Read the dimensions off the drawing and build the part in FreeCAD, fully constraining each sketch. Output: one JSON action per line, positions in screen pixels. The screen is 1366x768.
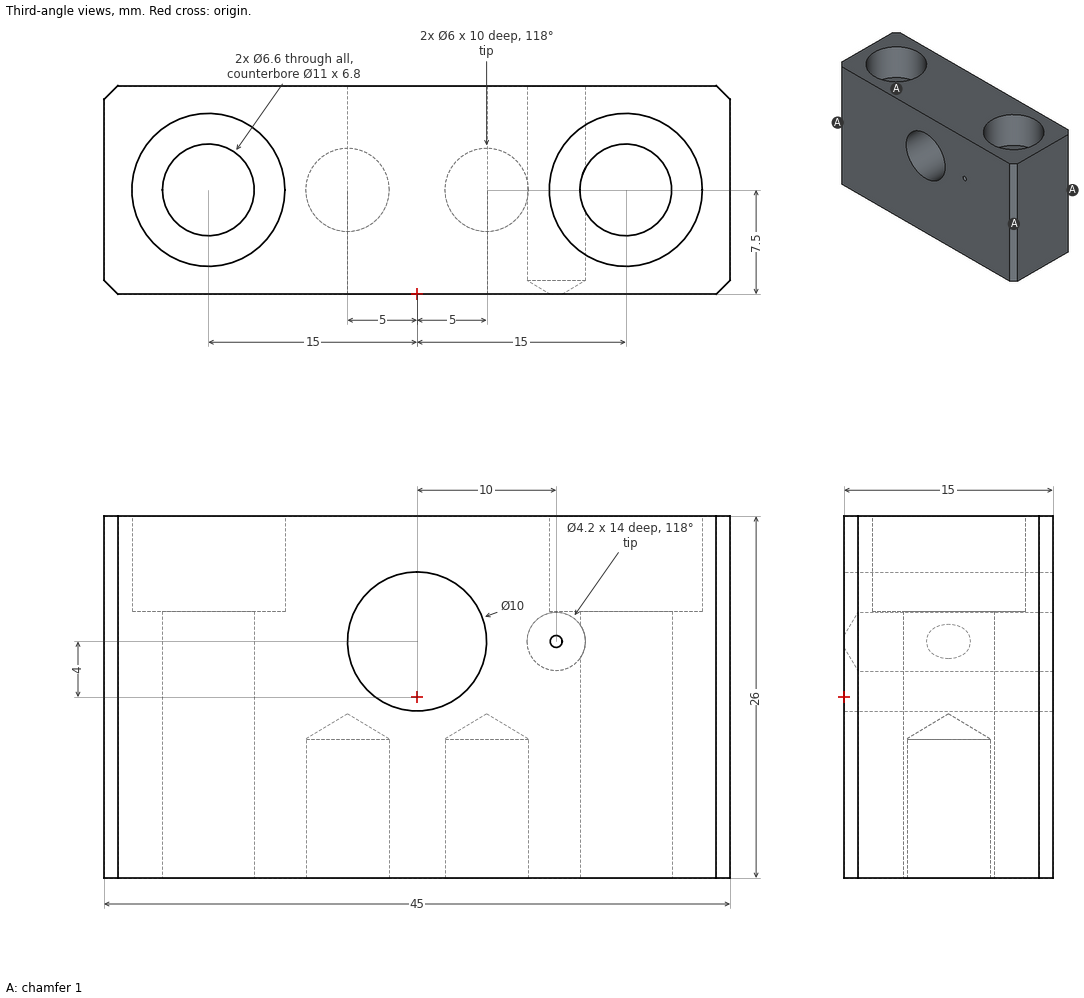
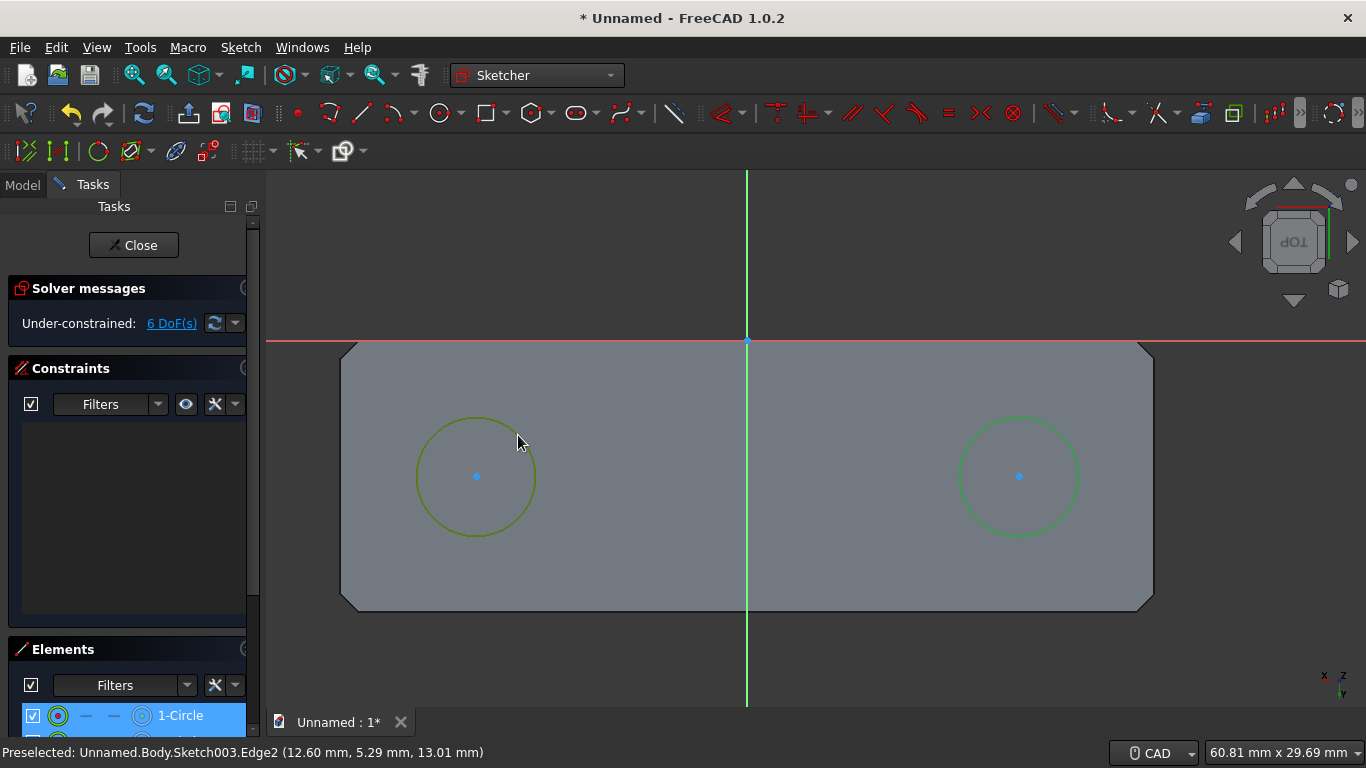
{"action": "left_click", "coordinate": [950, 114]}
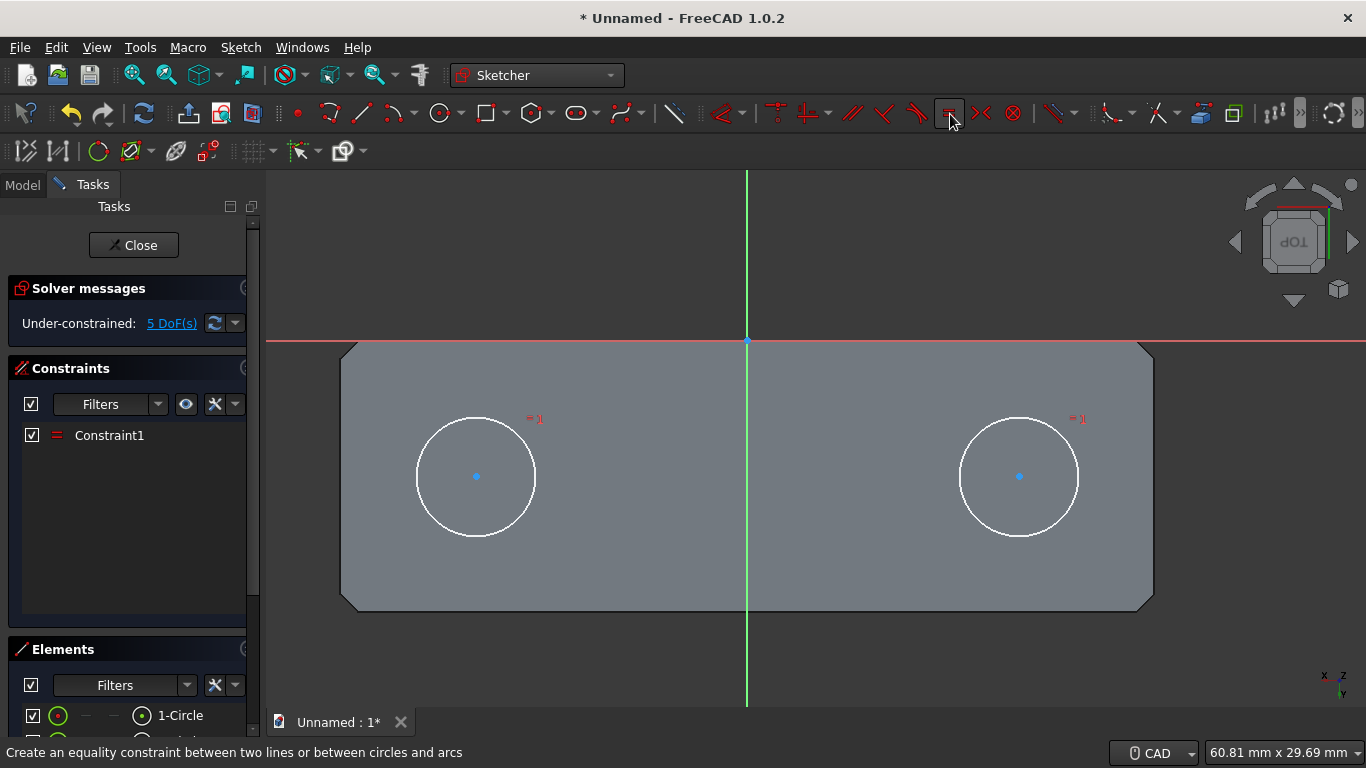
{"action": "left_click", "coordinate": [1019, 477]}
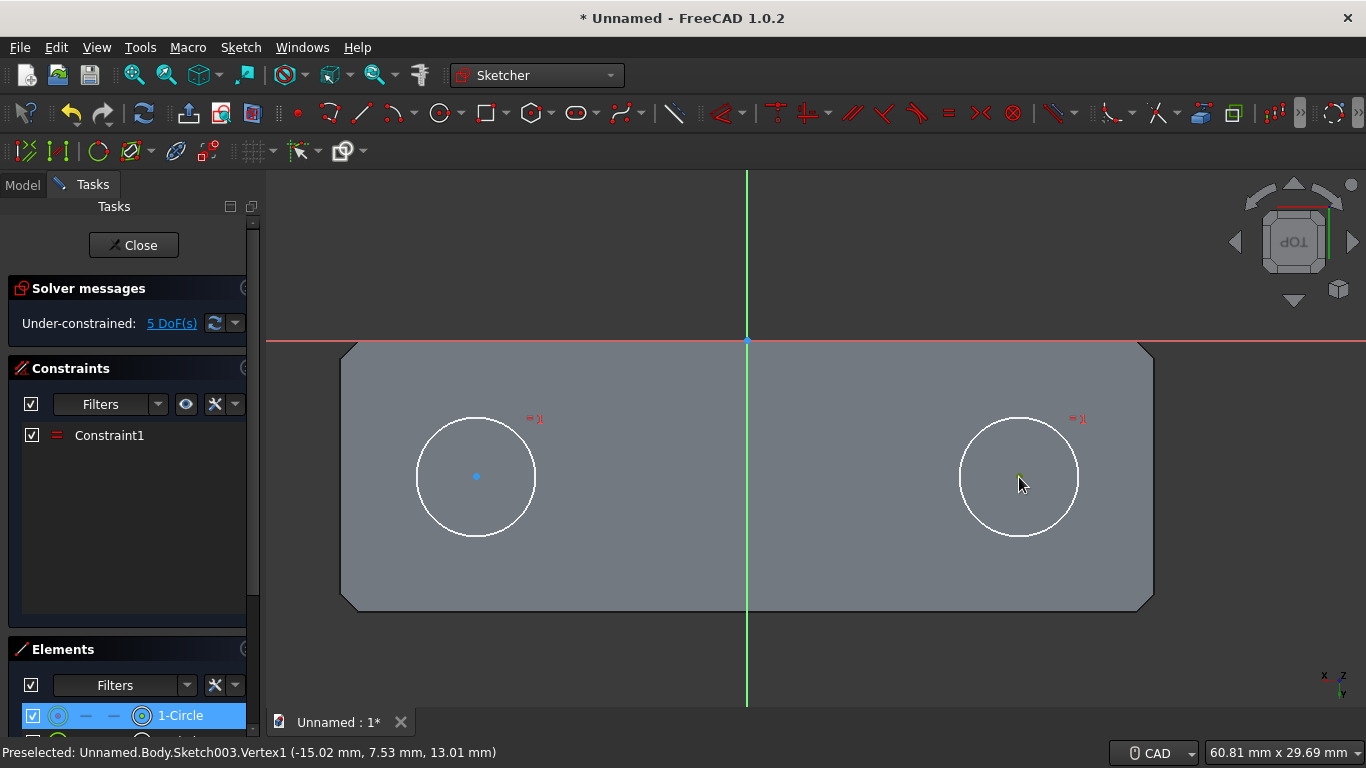
{"action": "left_click", "coordinate": [476, 477]}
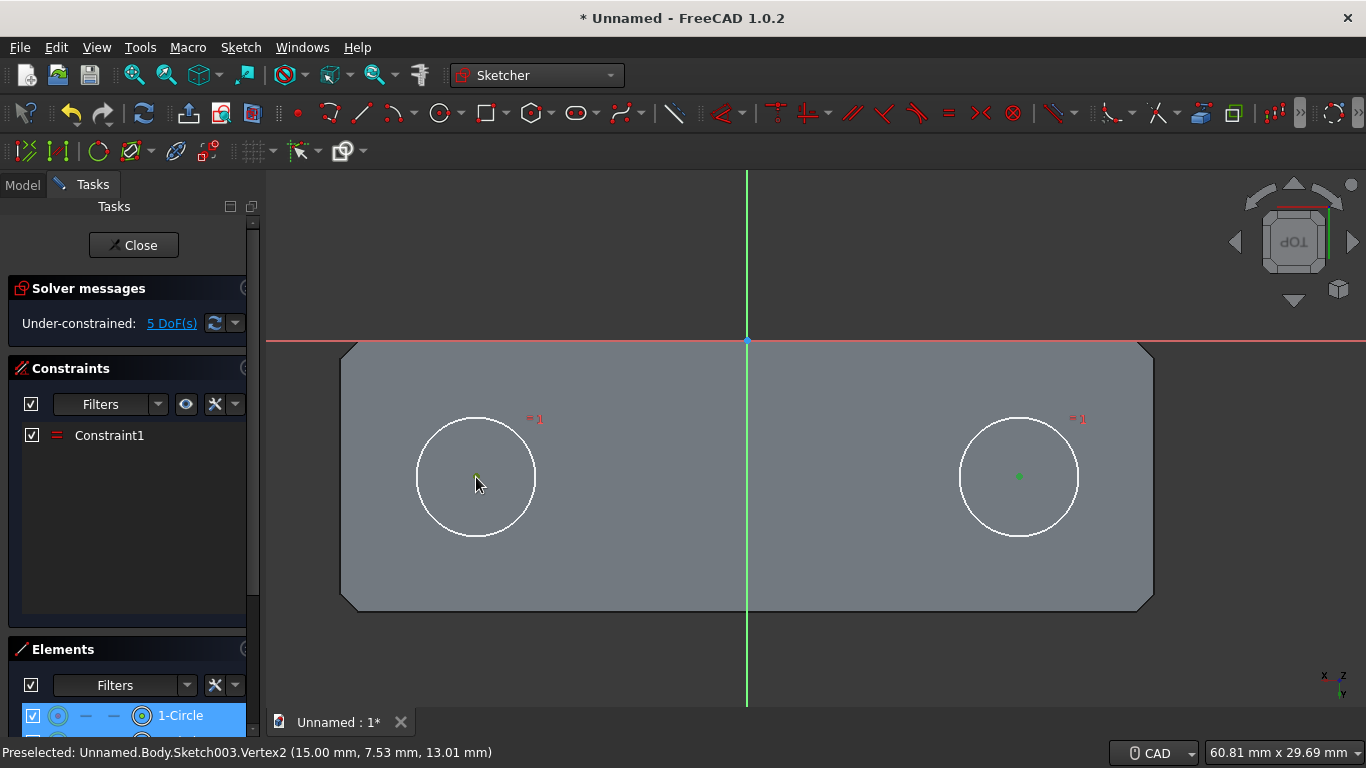
{"action": "left_click", "coordinate": [830, 114]}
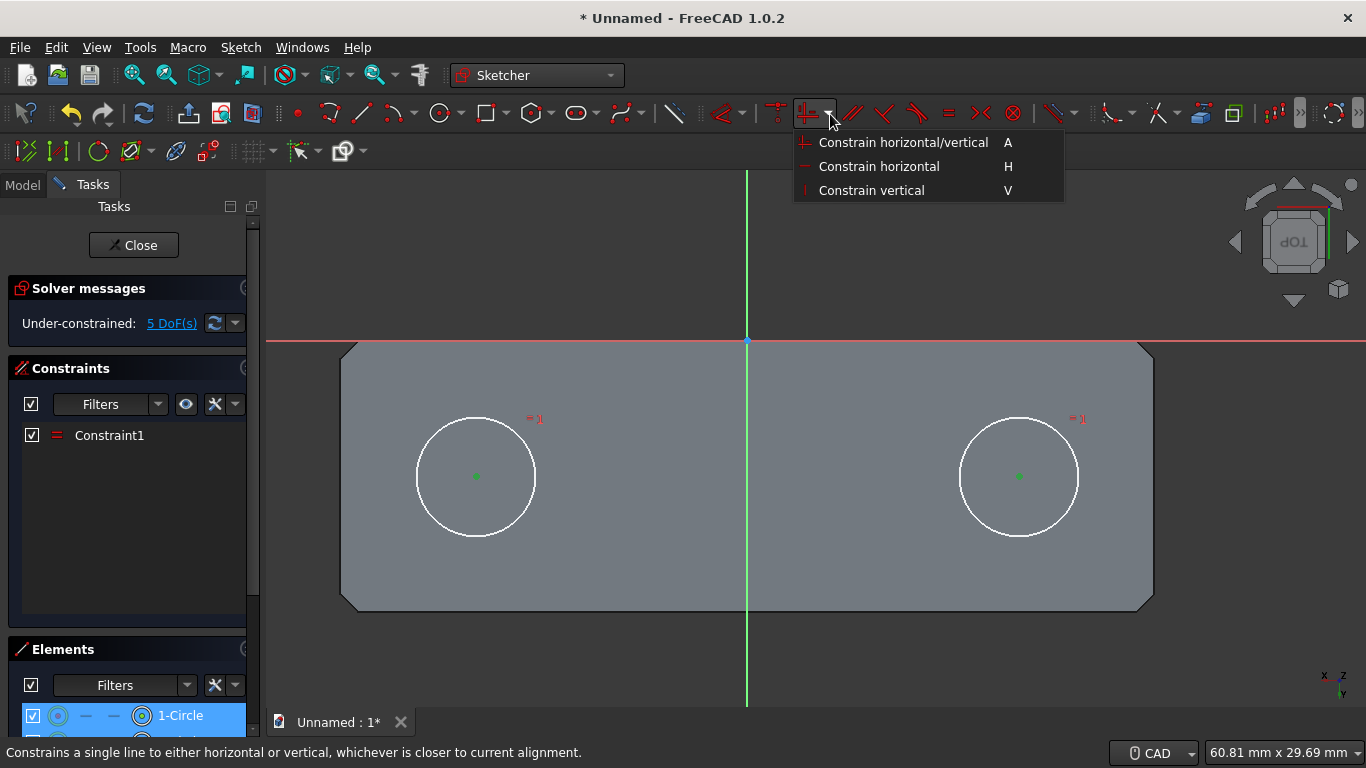
{"action": "left_click", "coordinate": [929, 166]}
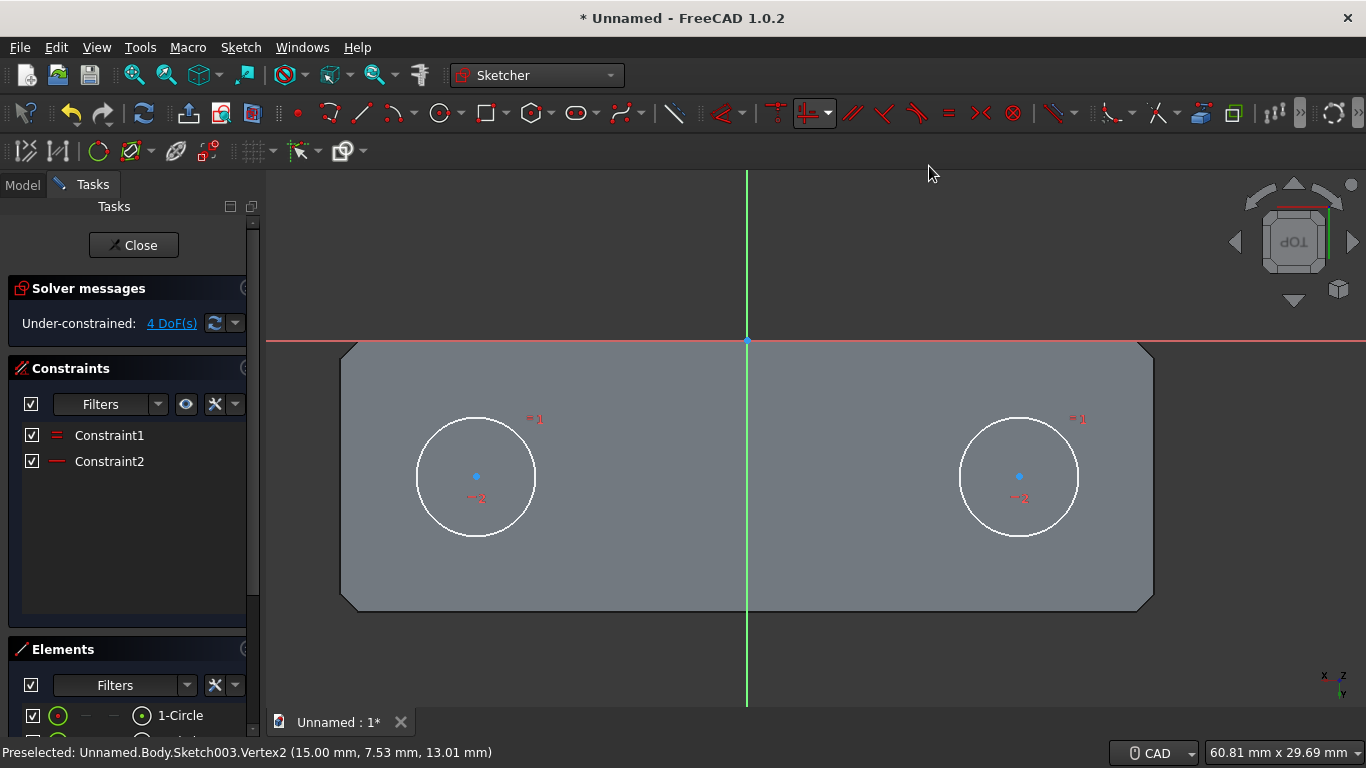
{"action": "left_click", "coordinate": [722, 114]}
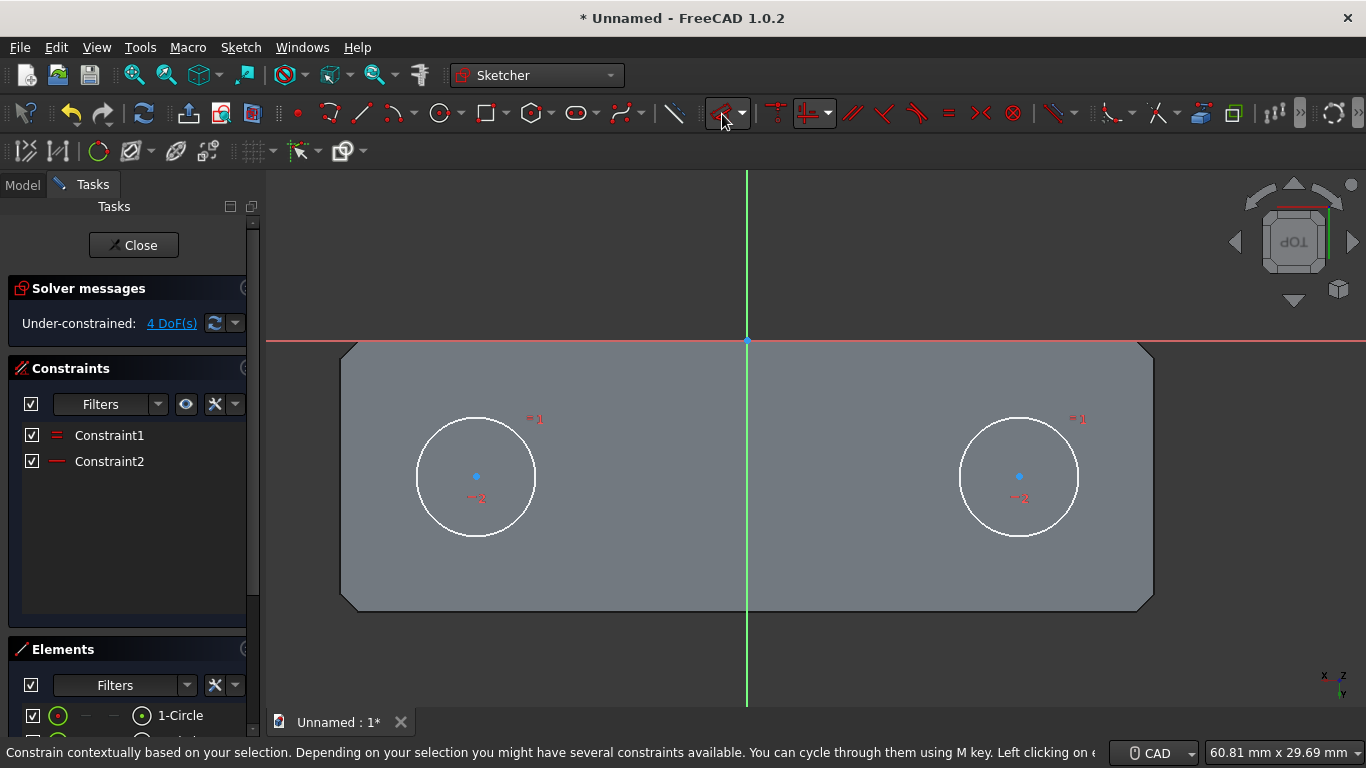
{"action": "left_click", "coordinate": [1061, 435]}
{"action": "left_click", "coordinate": [1084, 412]}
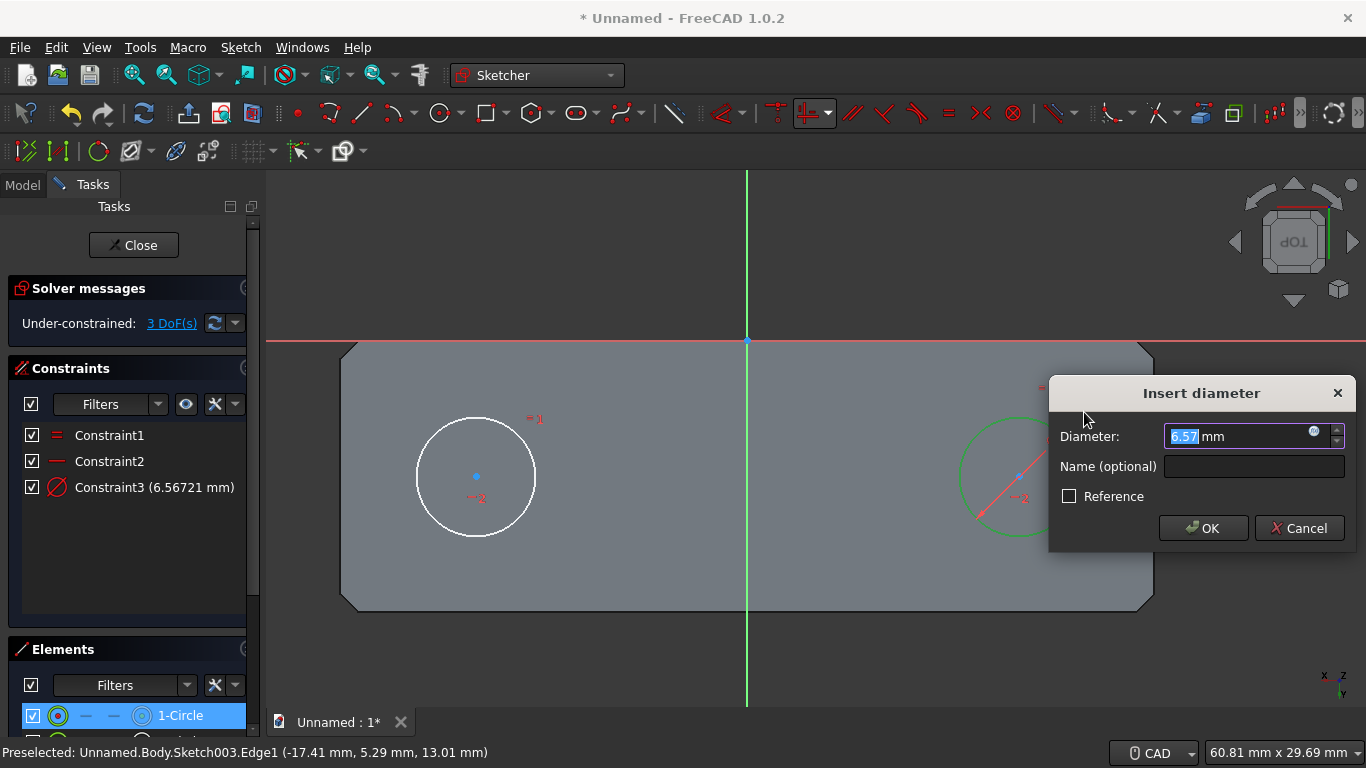
{"action": "type", "text": "6.6"}
{"action": "key", "text": "Return"}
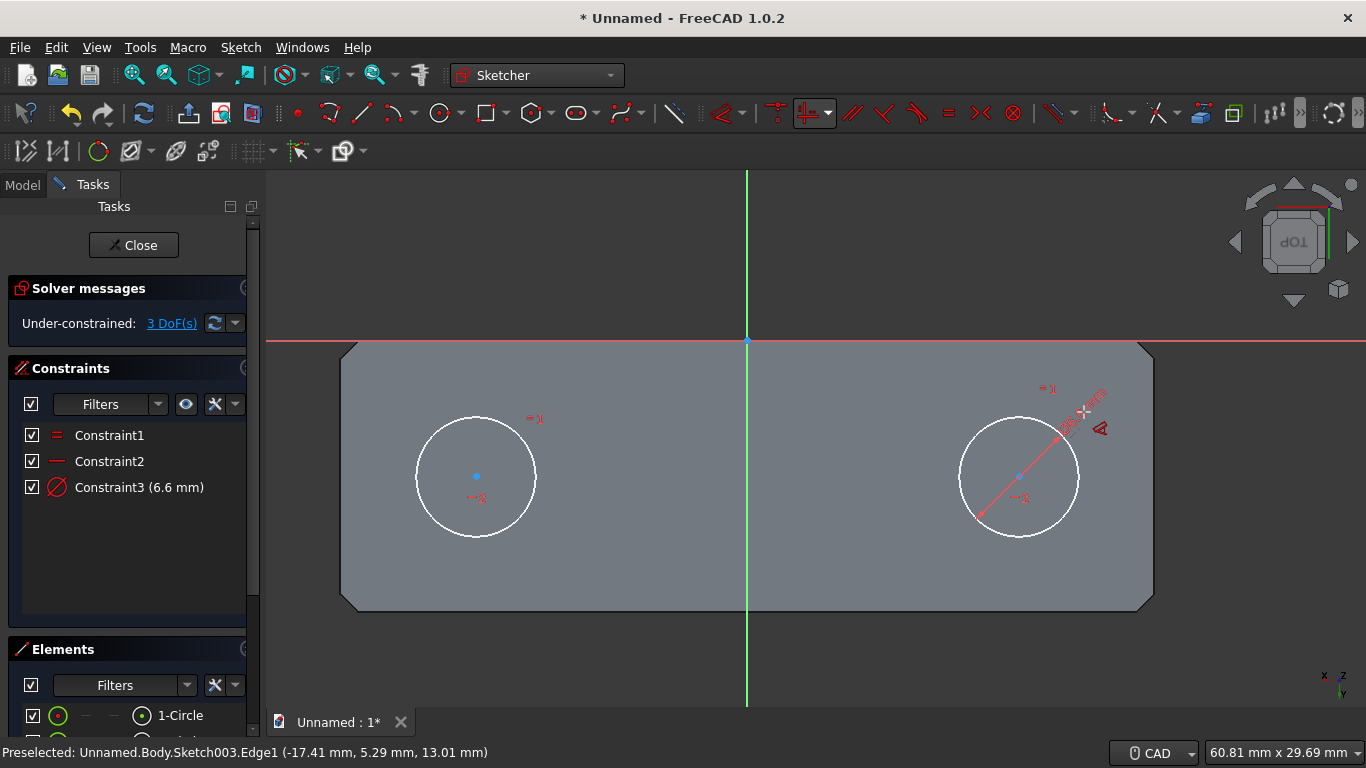
{"action": "left_click", "coordinate": [1019, 477]}
{"action": "left_click", "coordinate": [883, 307]}